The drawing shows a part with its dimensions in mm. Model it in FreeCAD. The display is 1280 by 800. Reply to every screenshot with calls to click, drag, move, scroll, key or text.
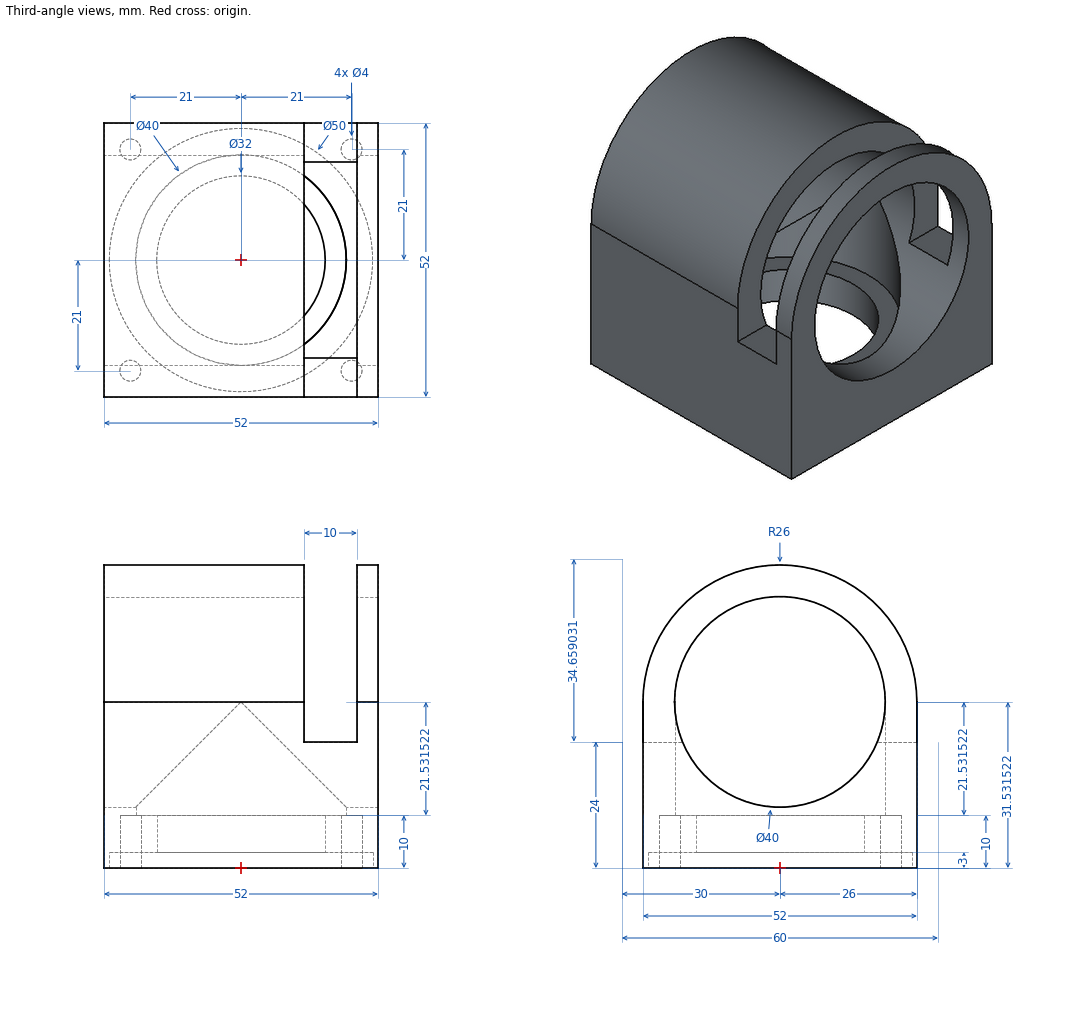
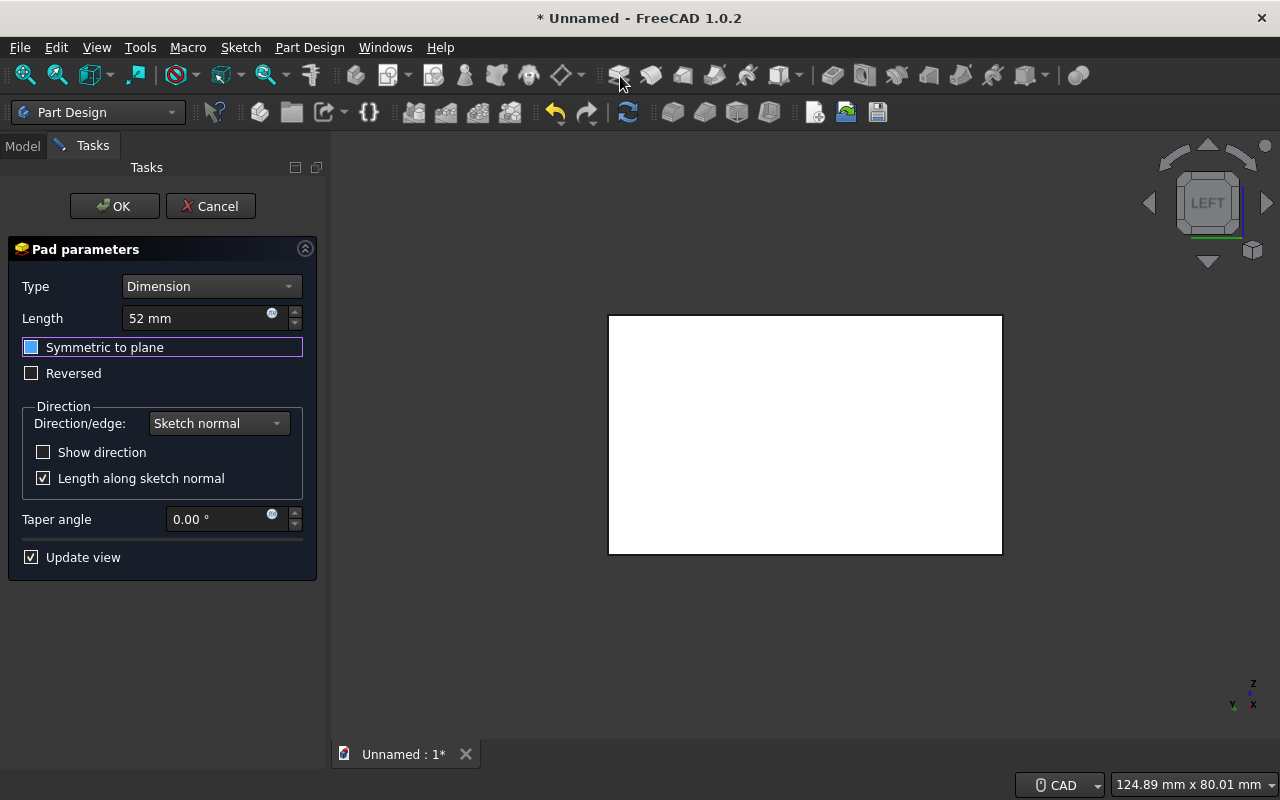
click(30, 373)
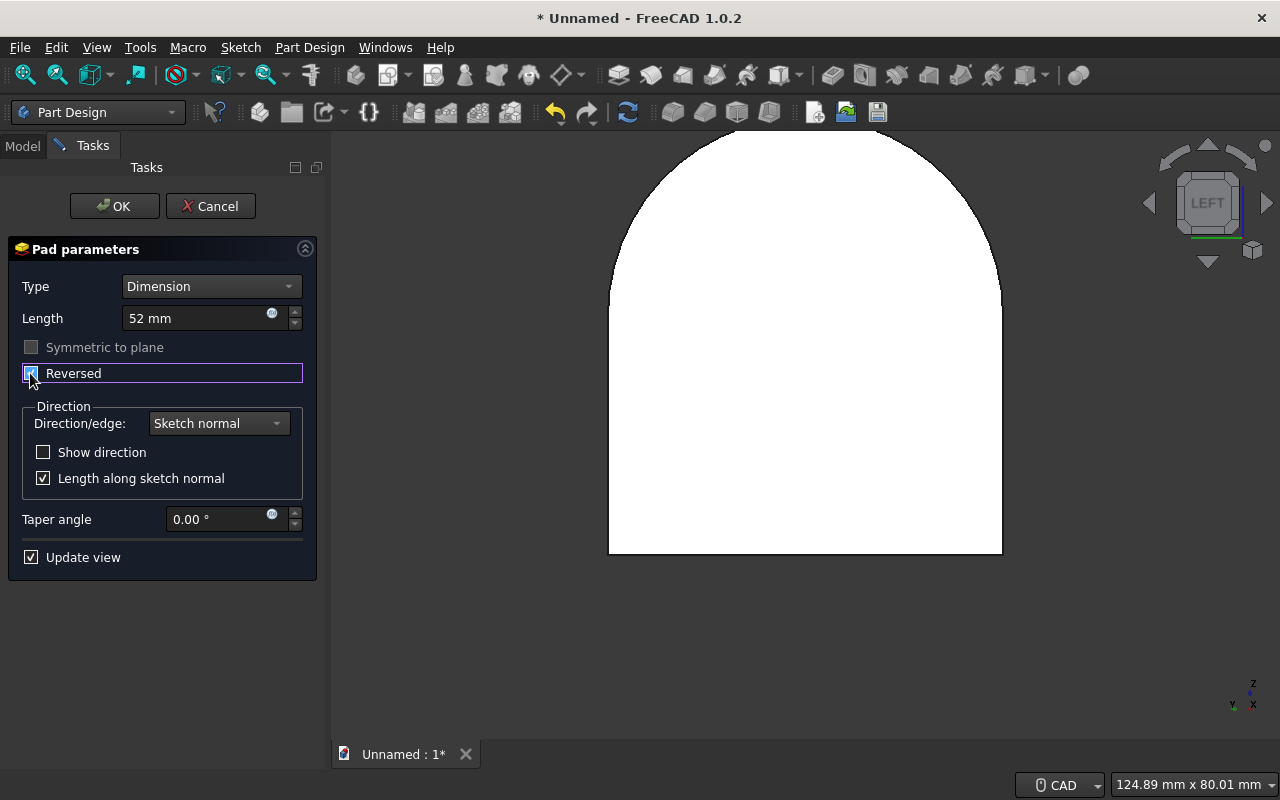
click(115, 206)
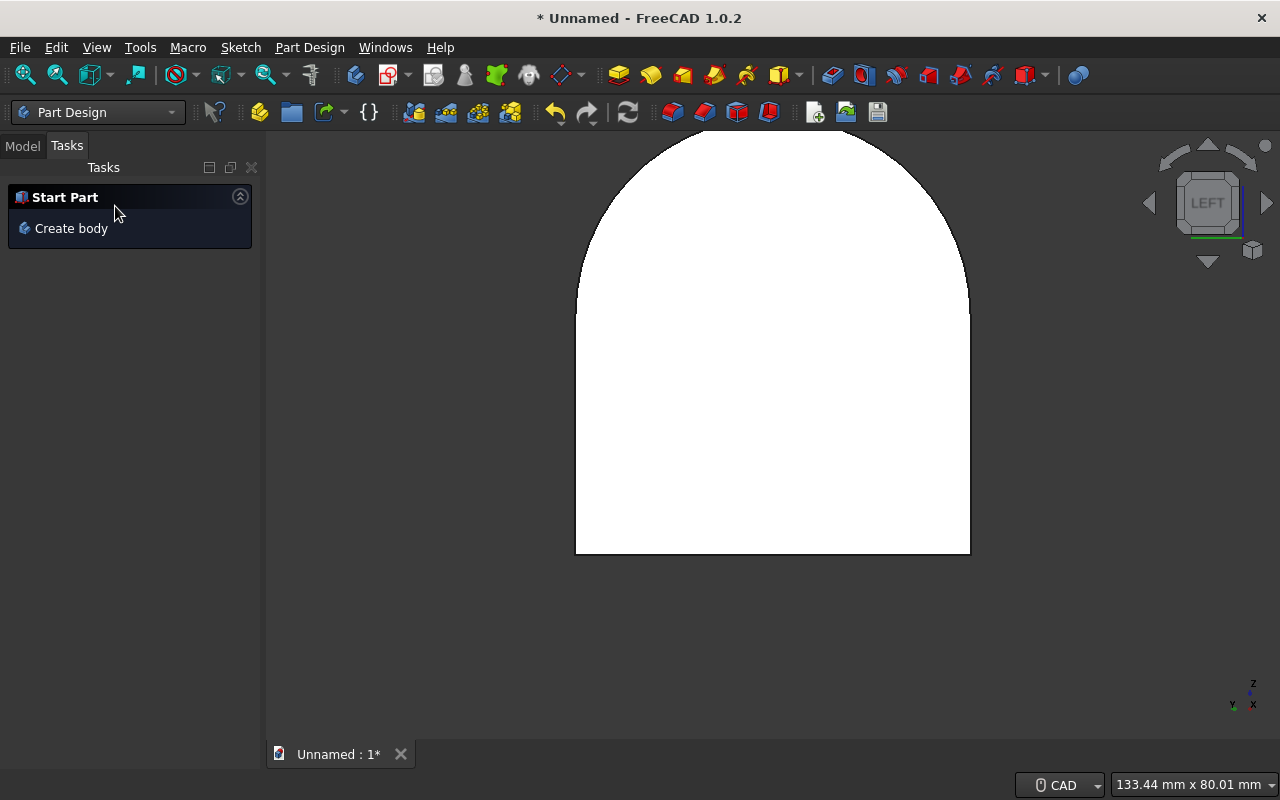
click(26, 76)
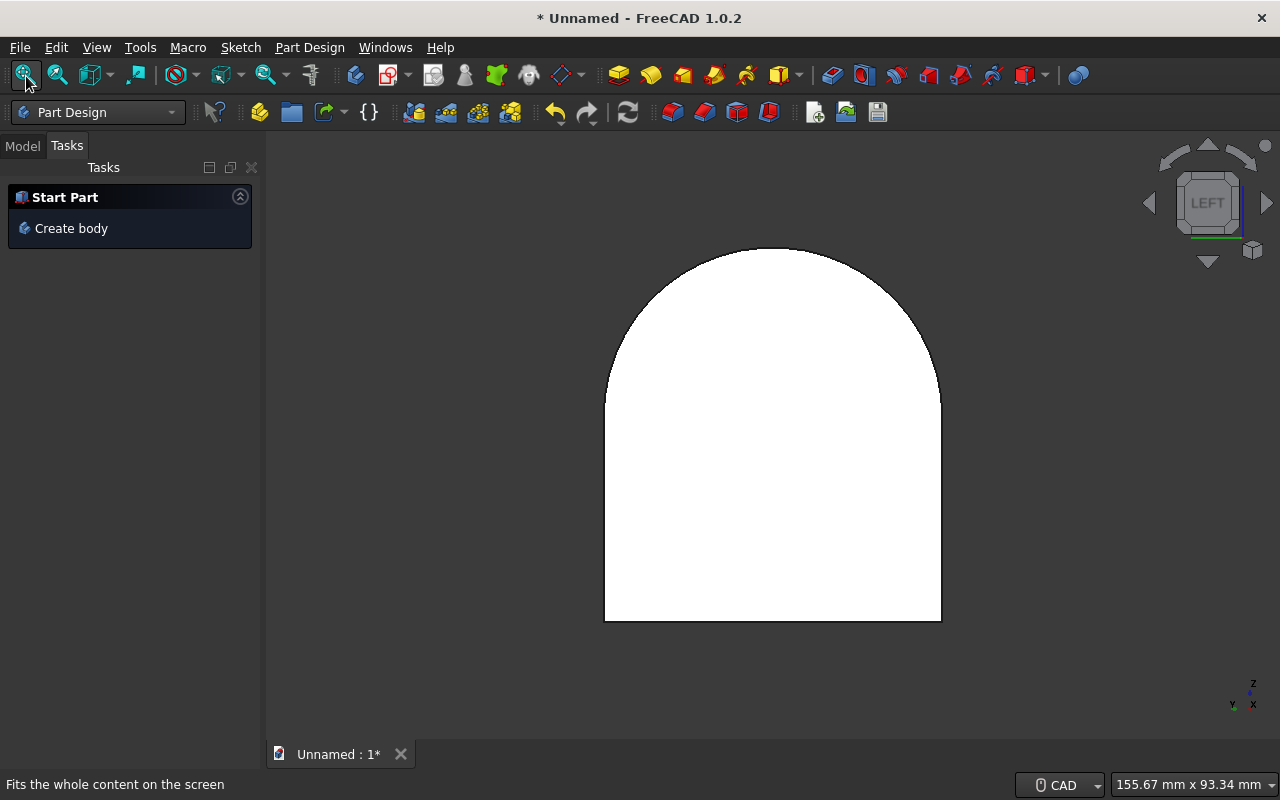
click(773, 434)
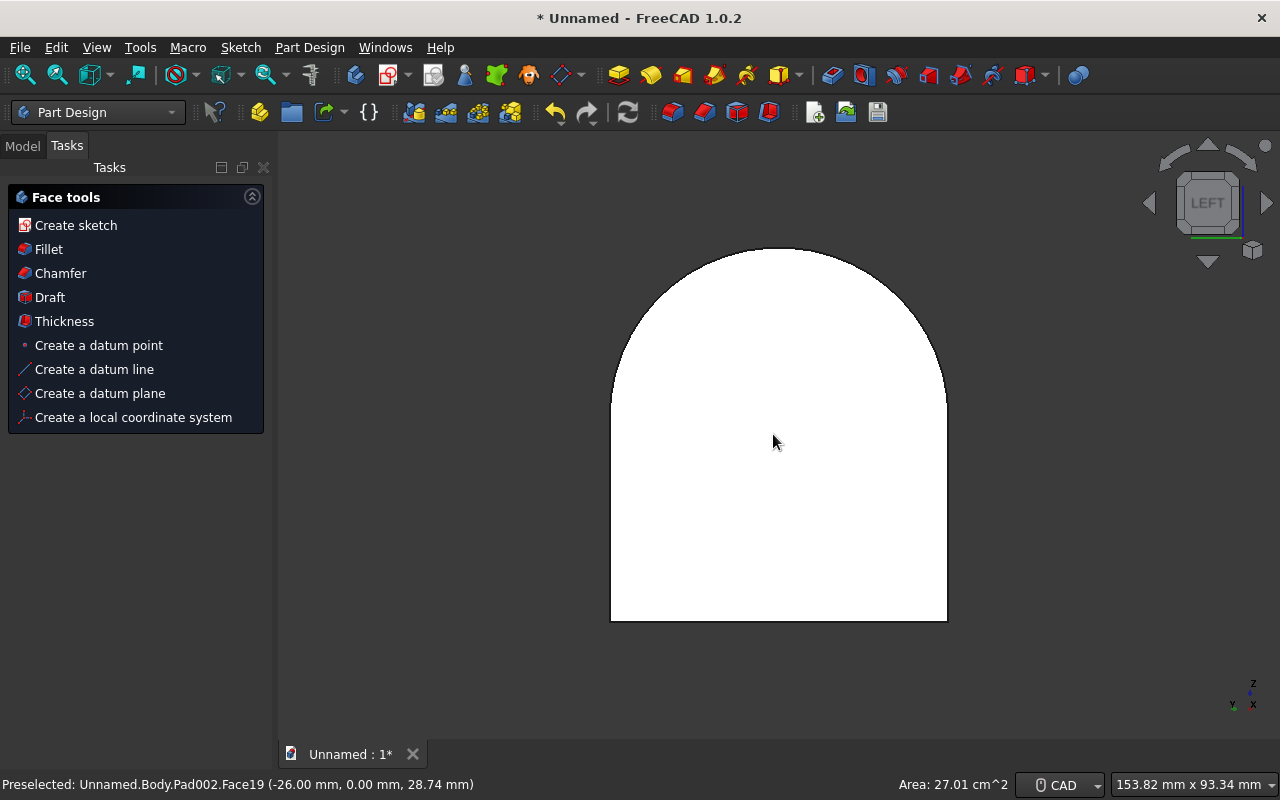
click(388, 76)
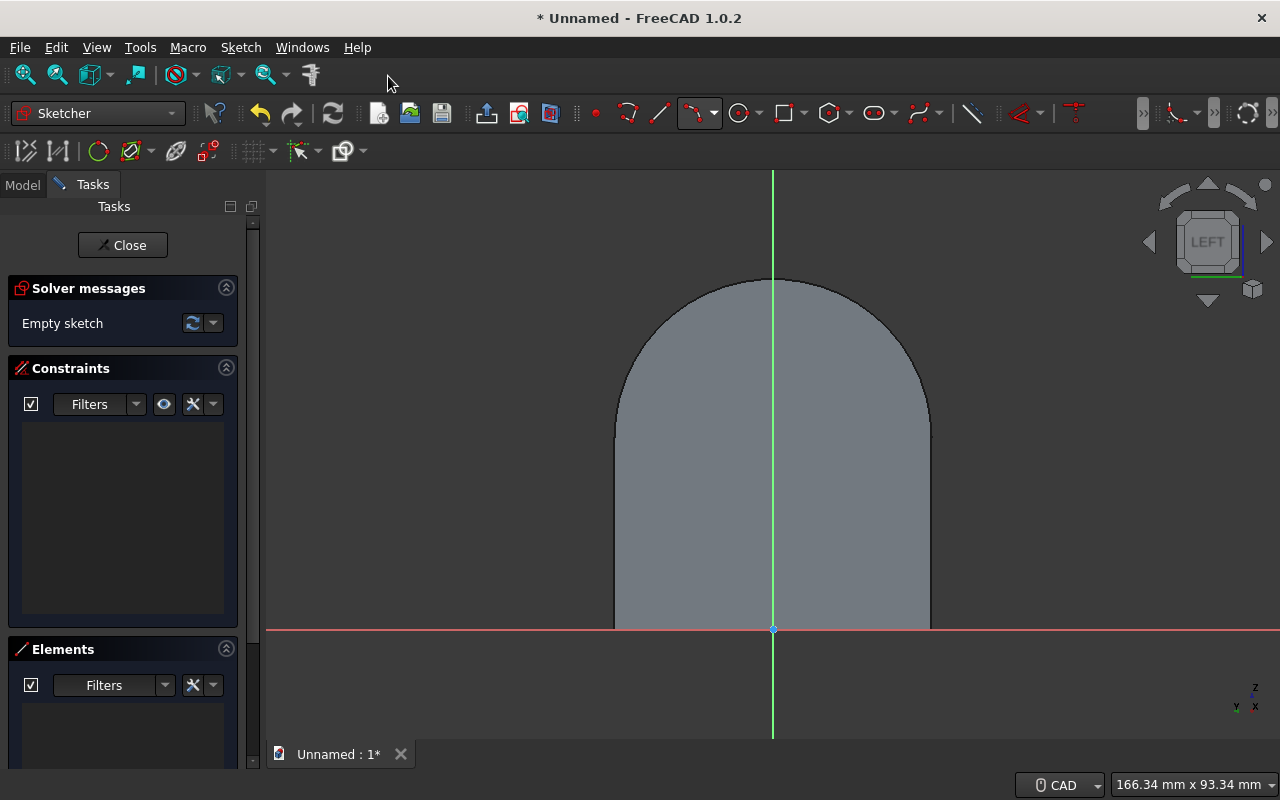
click(740, 114)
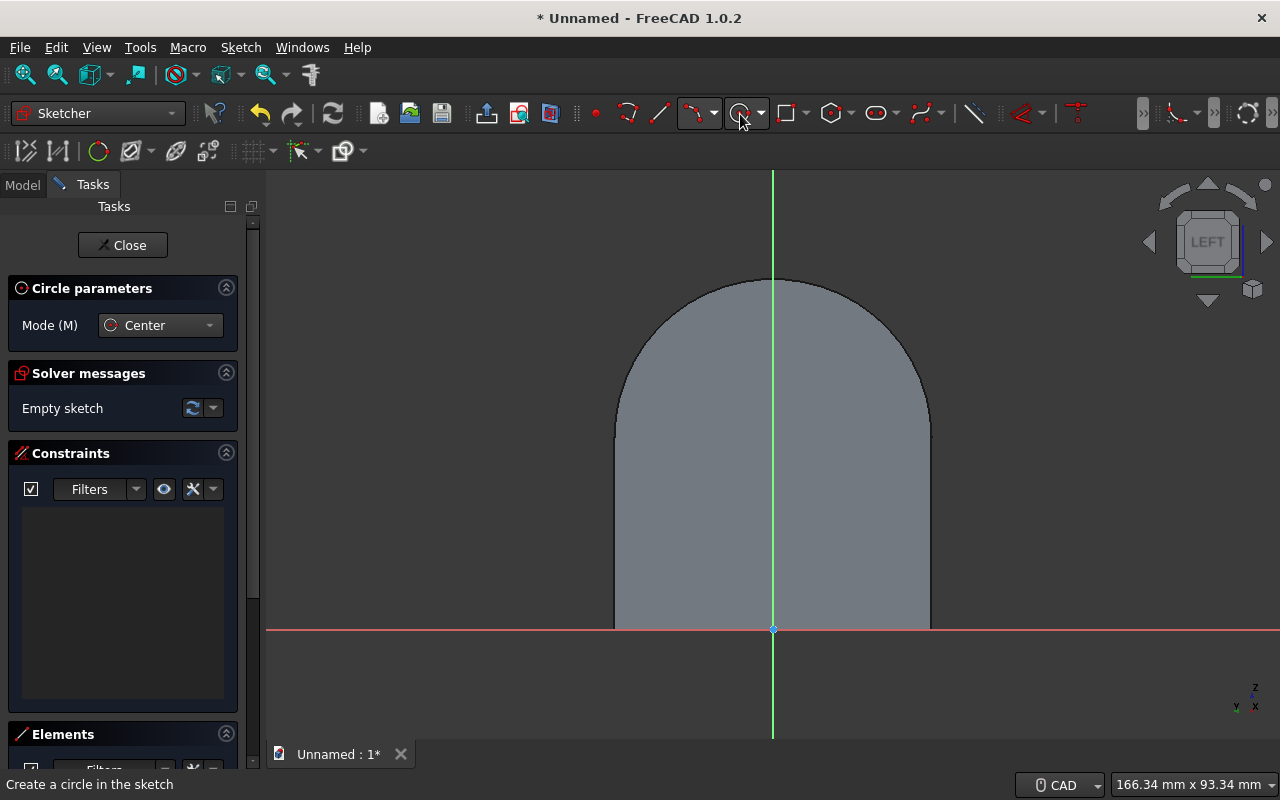
click(773, 437)
click(859, 351)
key(Escape)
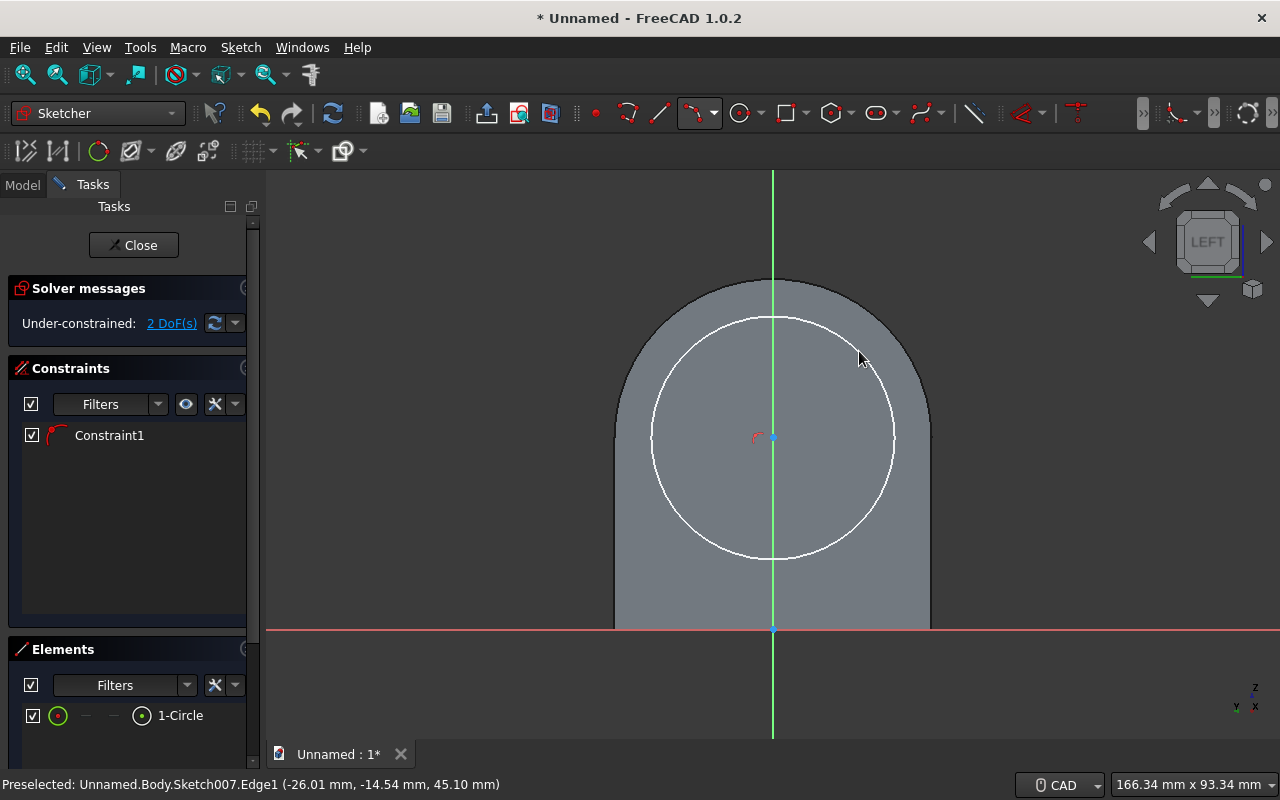
click(1022, 114)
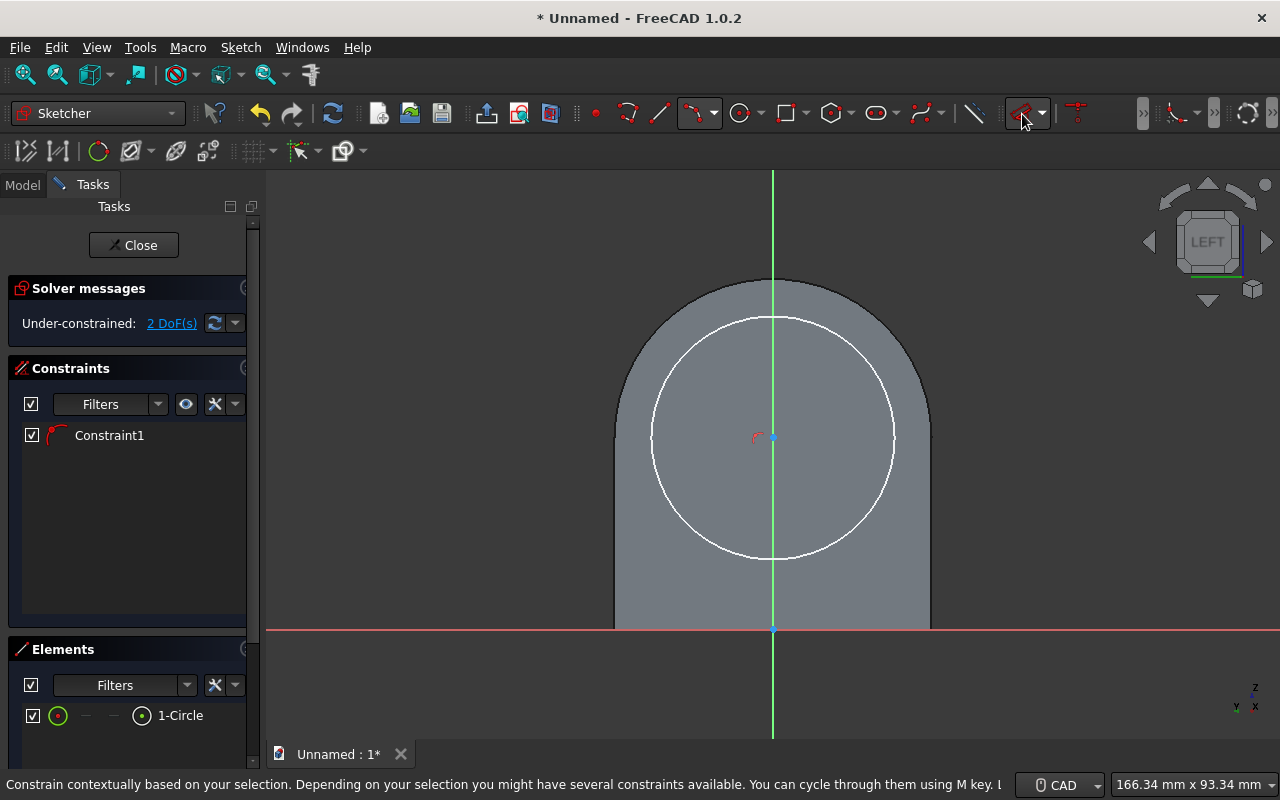
click(859, 352)
click(882, 329)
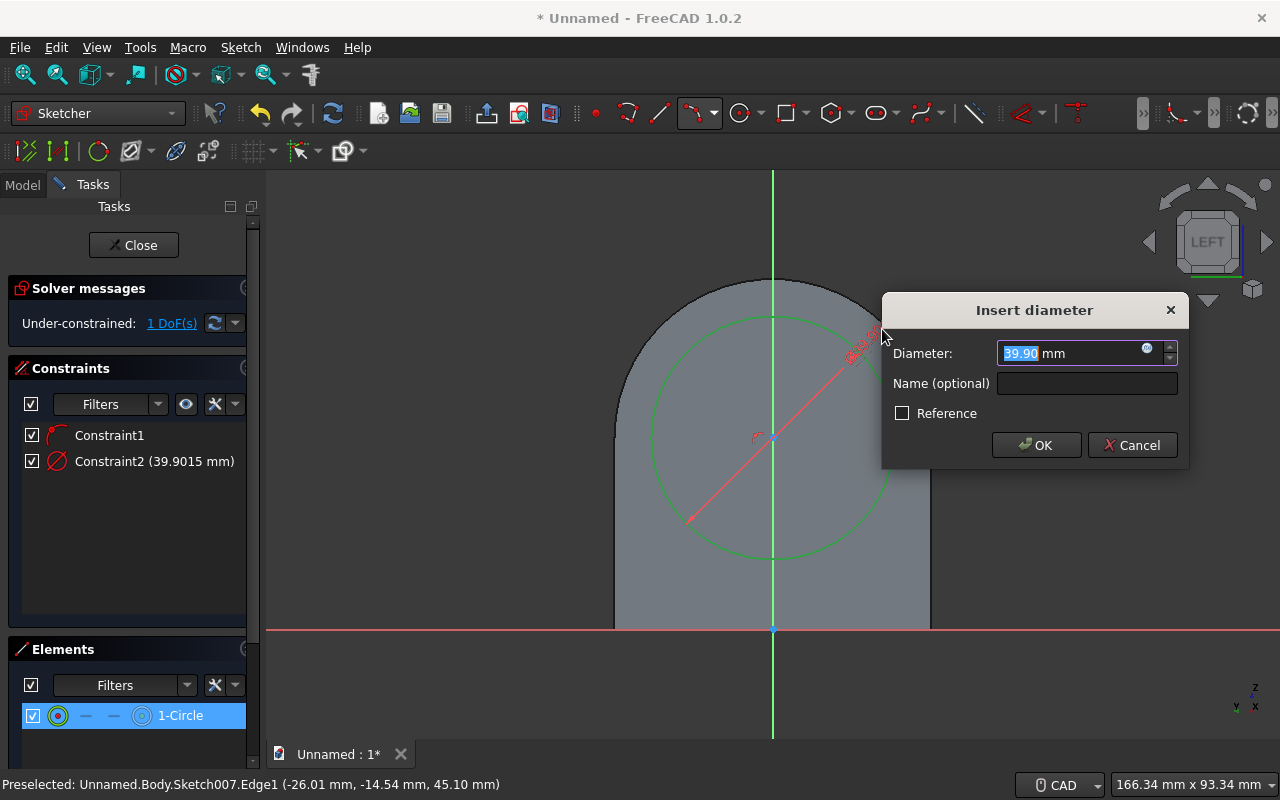
text(40)
key(Return)